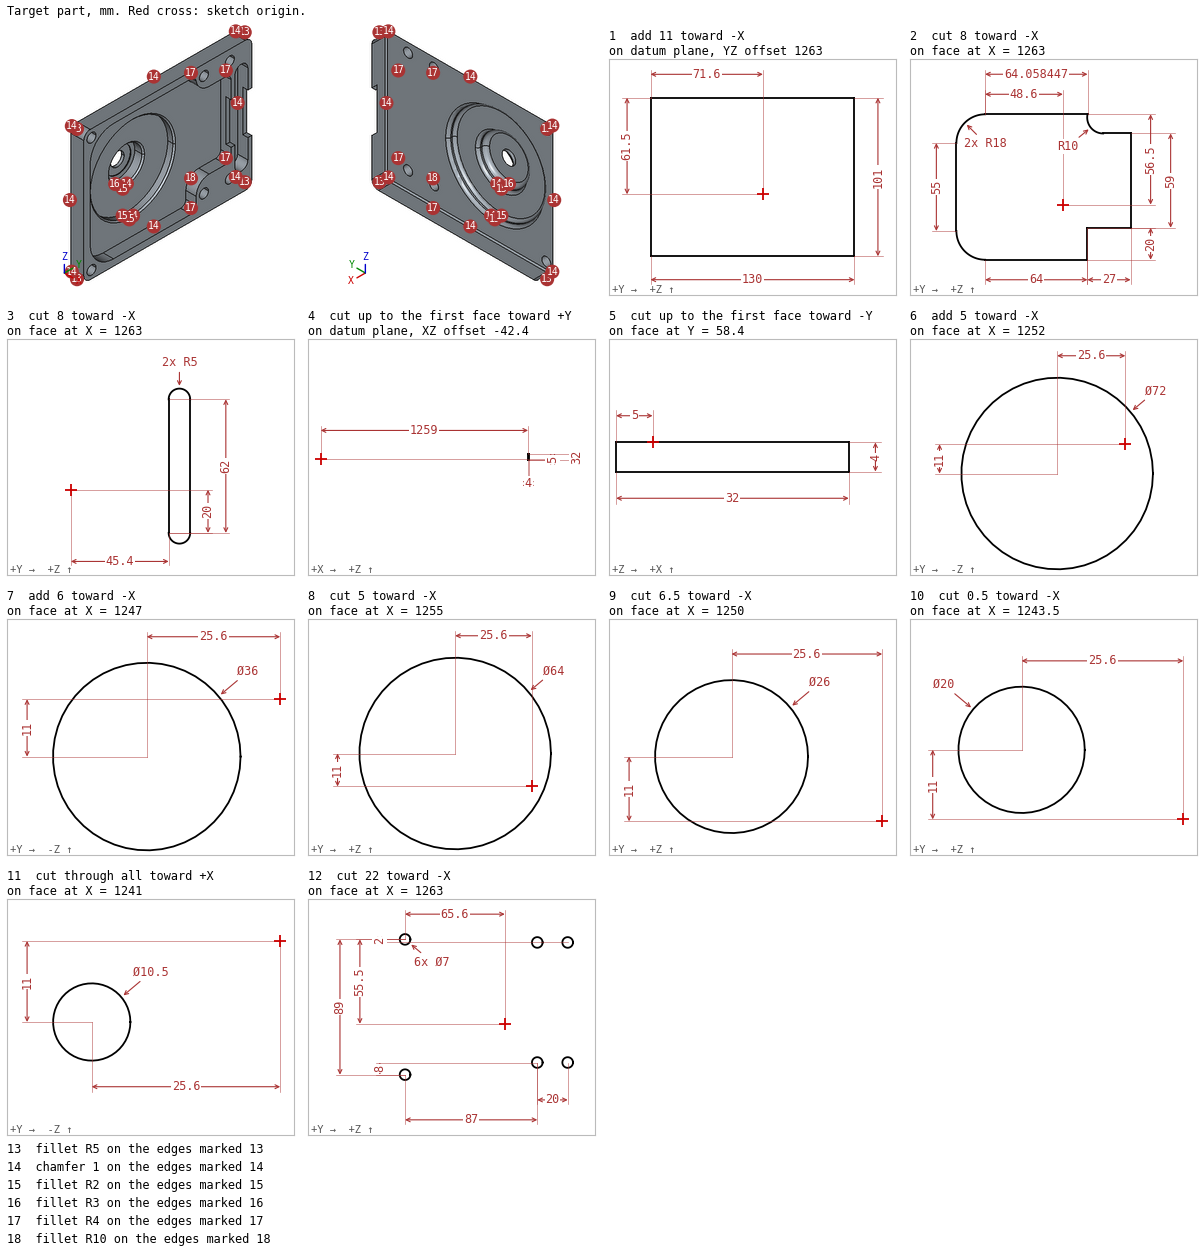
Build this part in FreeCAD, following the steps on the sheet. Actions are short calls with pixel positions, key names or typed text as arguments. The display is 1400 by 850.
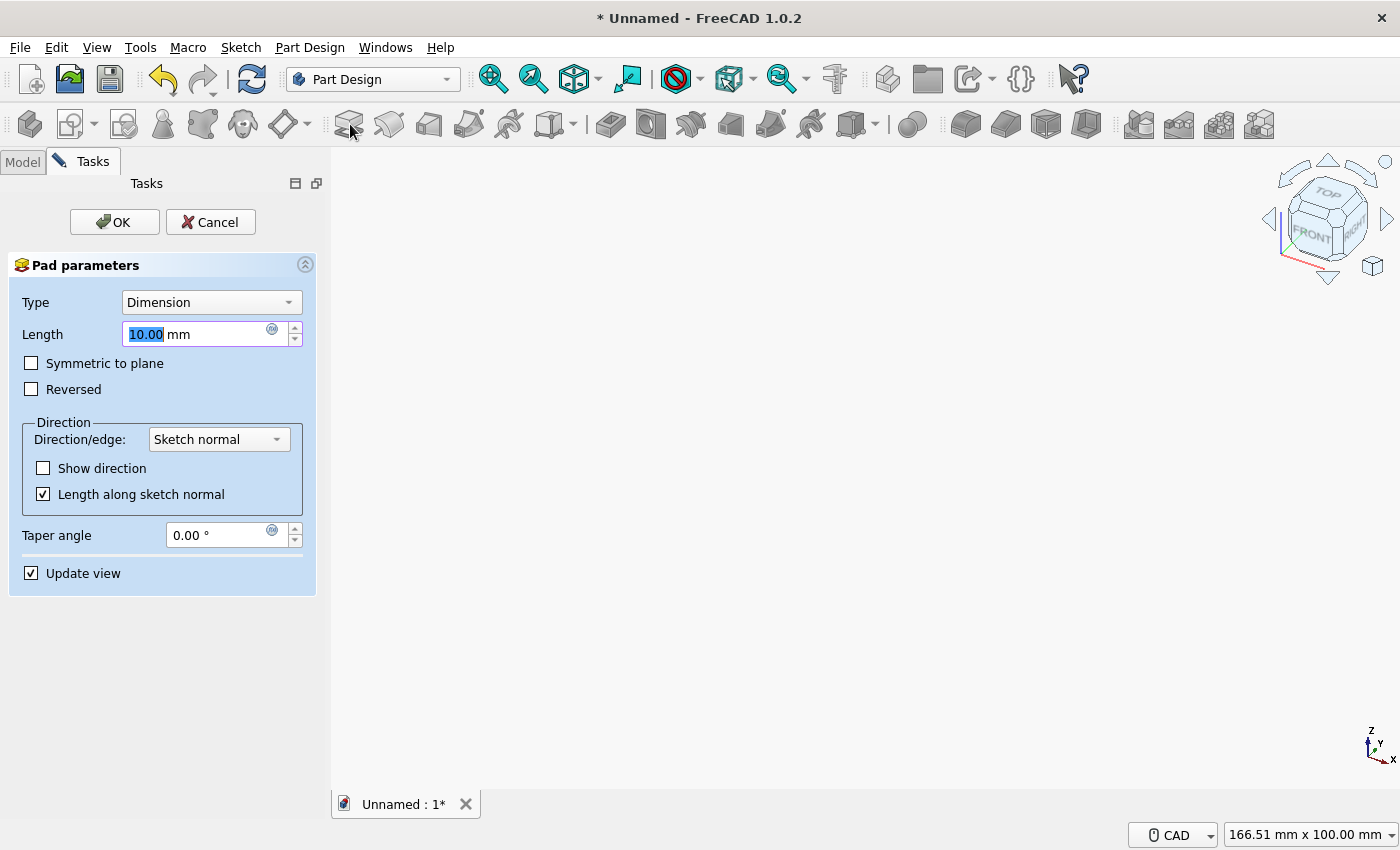
text(11)
key(Tab)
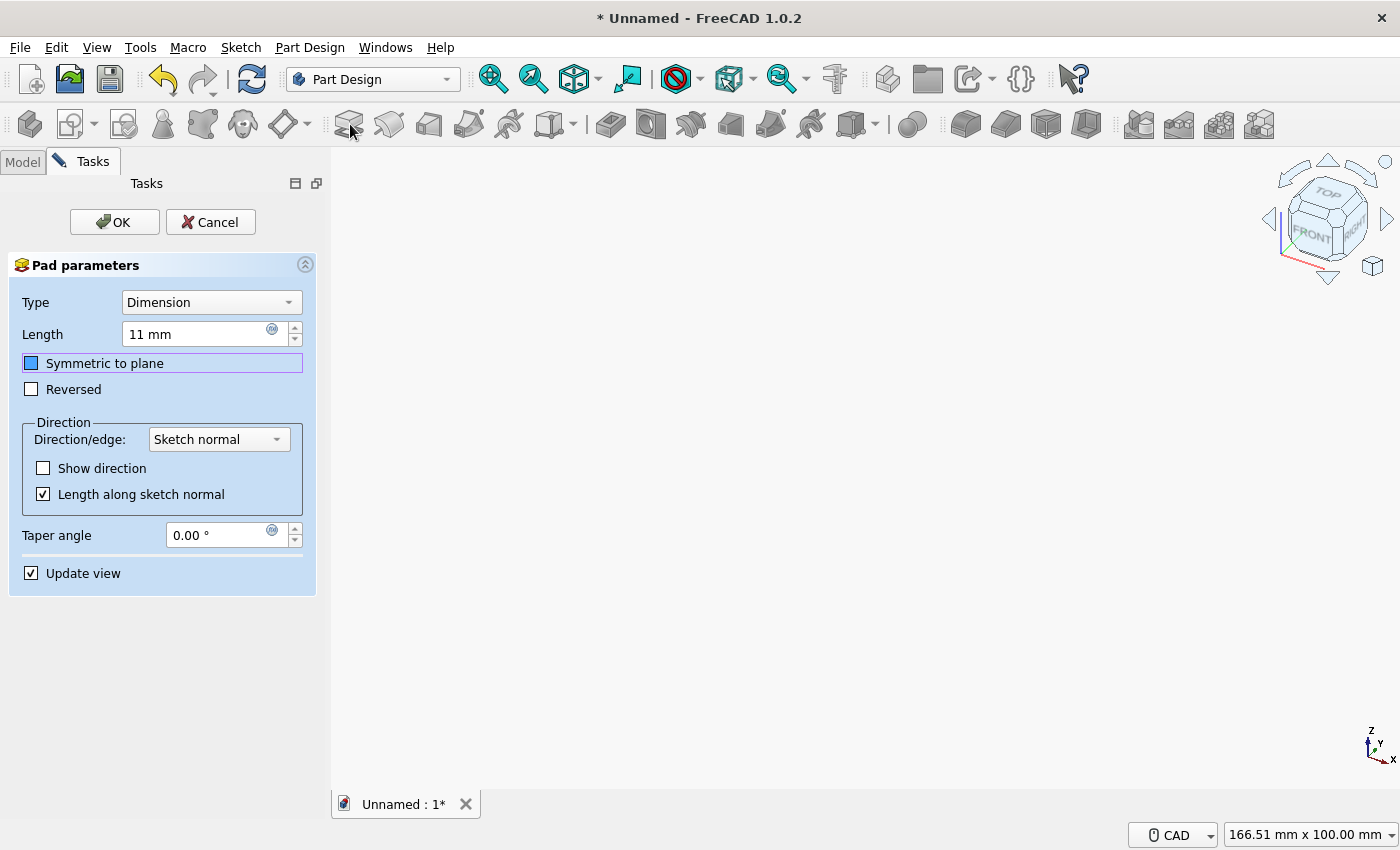
click(30, 389)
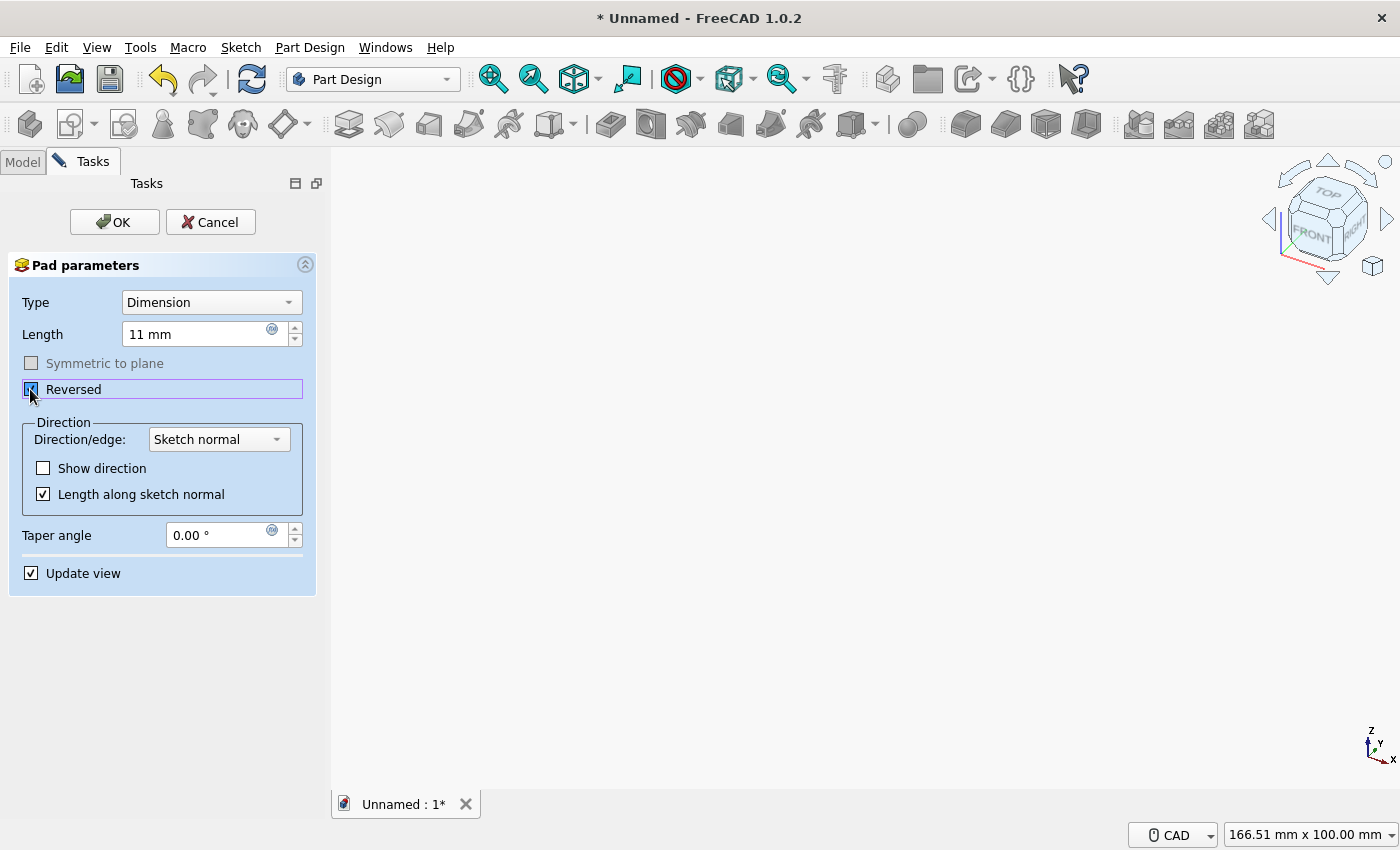
click(115, 222)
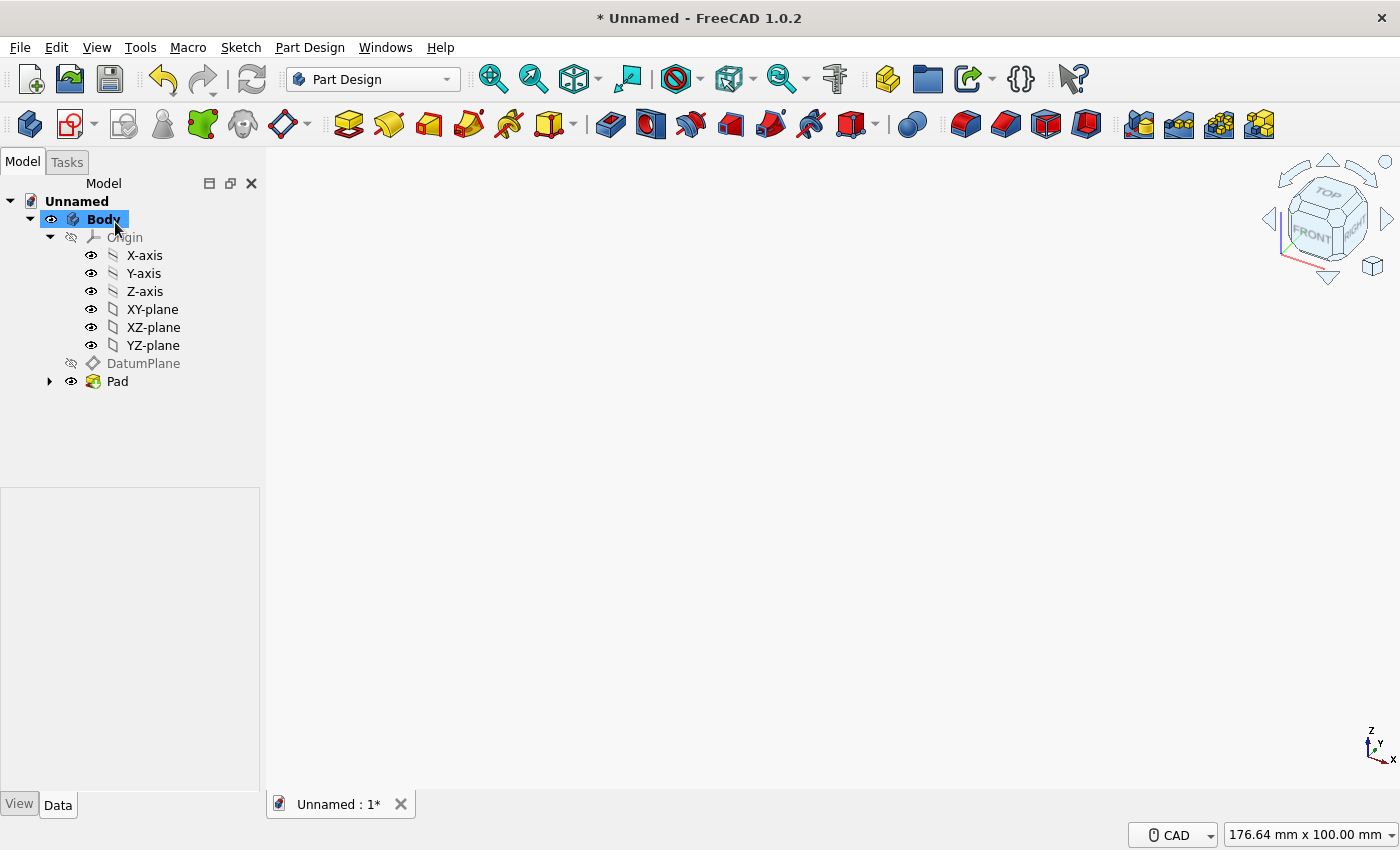
key(v)
key(f)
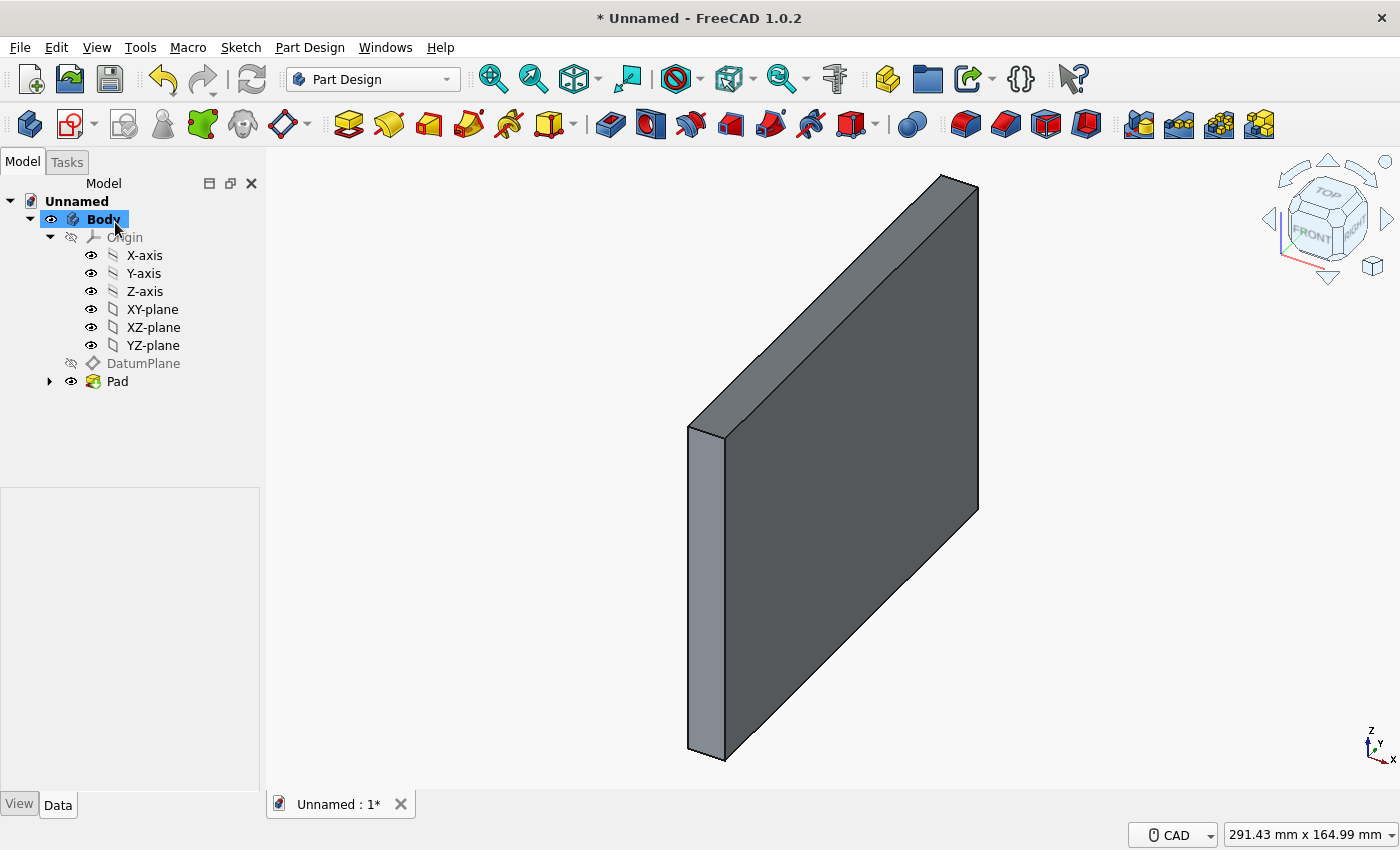
click(852, 473)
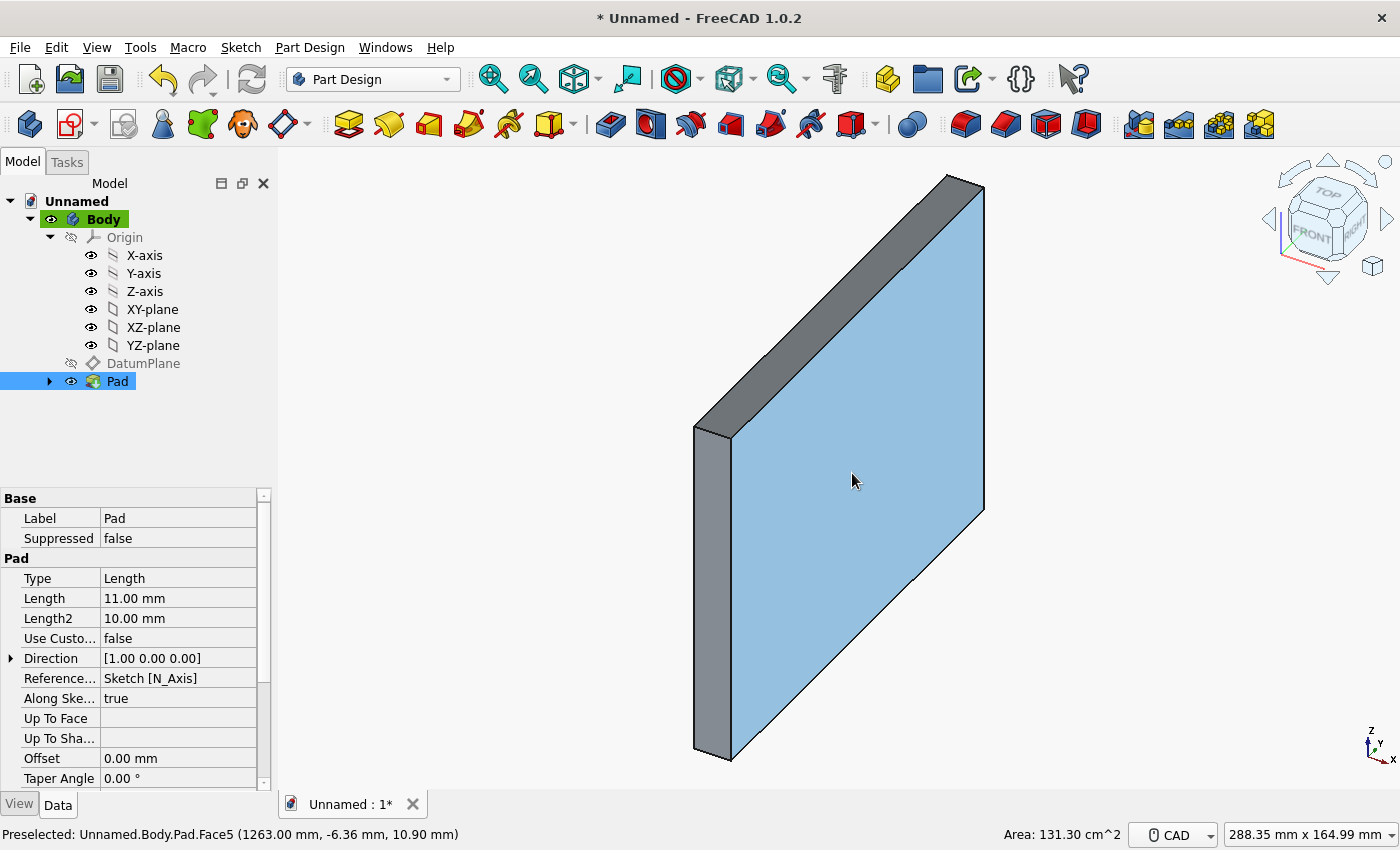
click(70, 124)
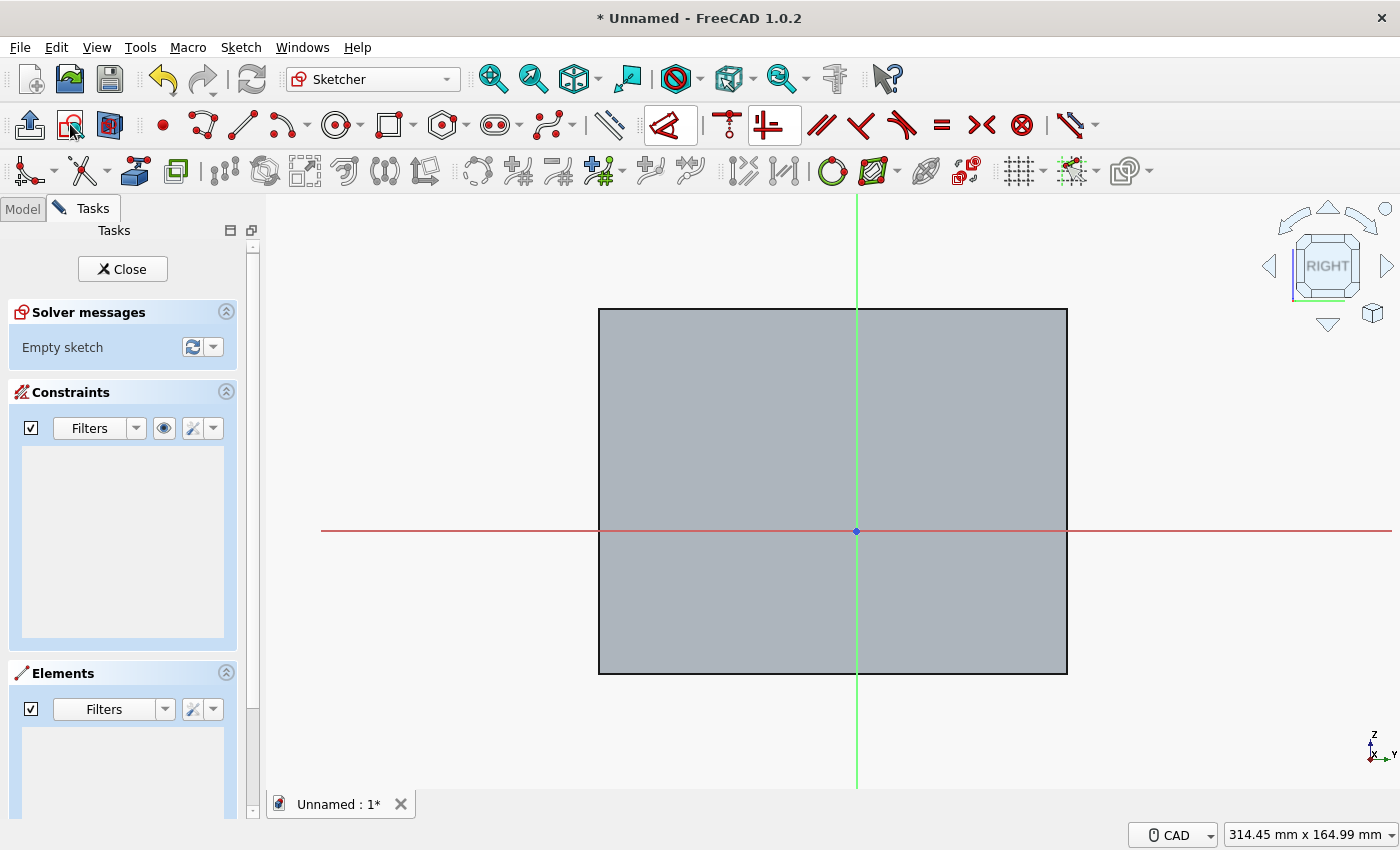
key(g)
key(l)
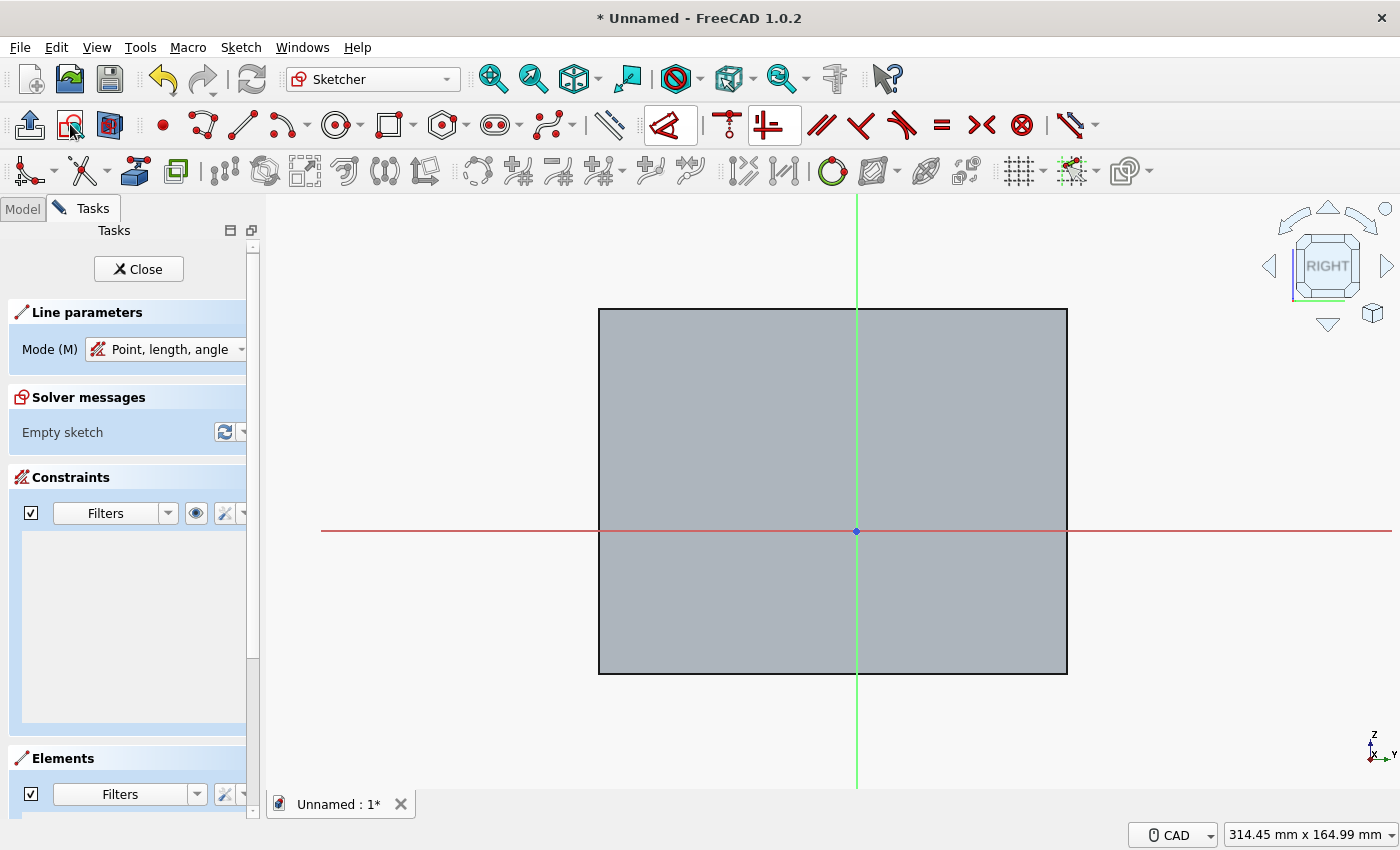
click(913, 327)
click(682, 327)